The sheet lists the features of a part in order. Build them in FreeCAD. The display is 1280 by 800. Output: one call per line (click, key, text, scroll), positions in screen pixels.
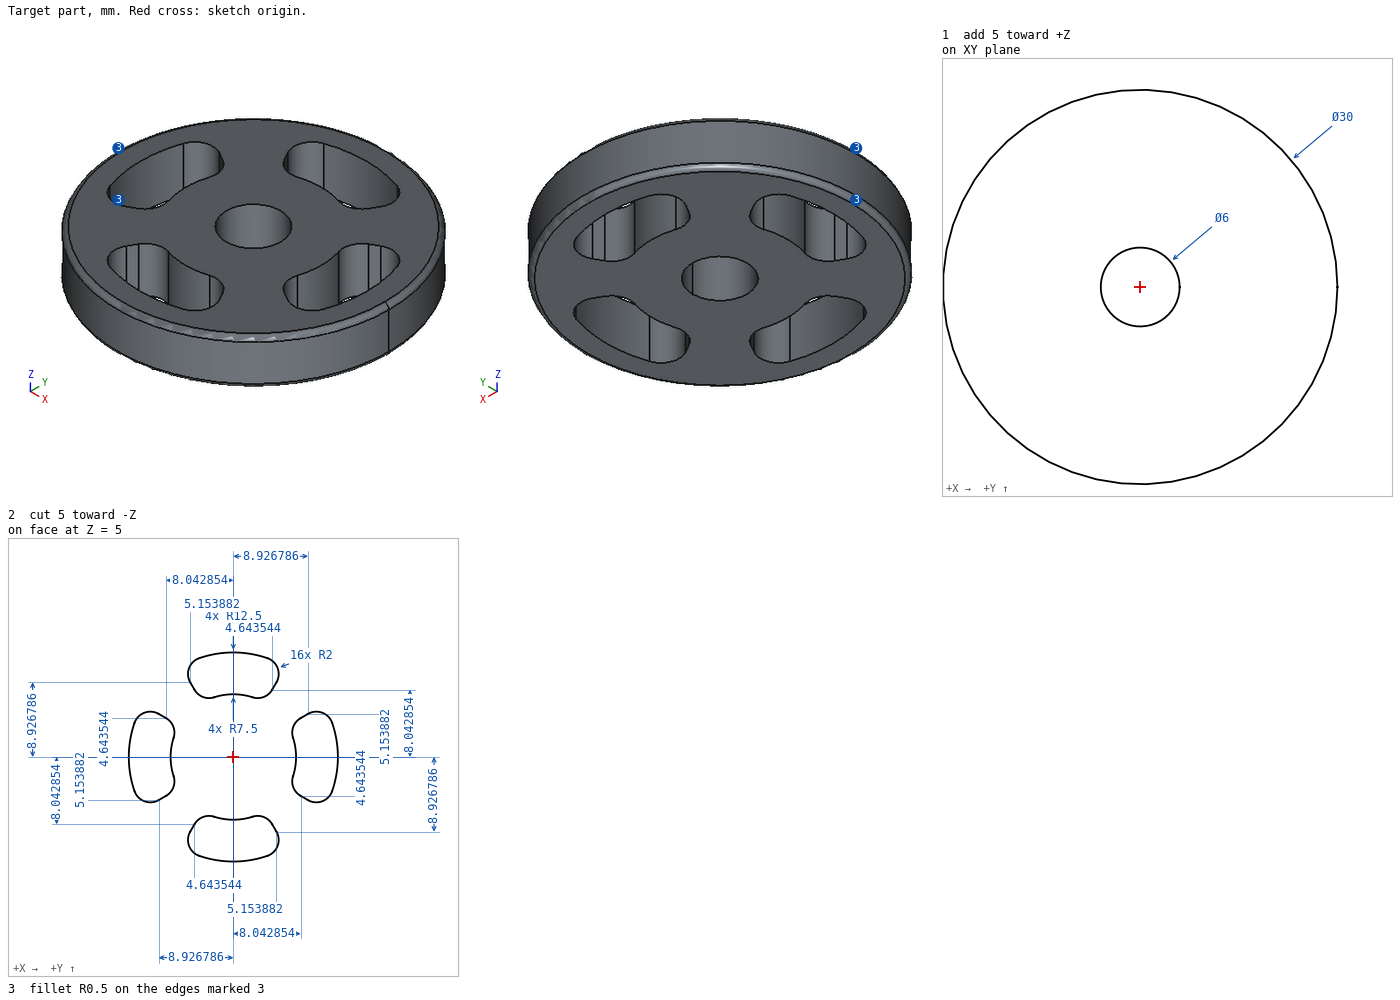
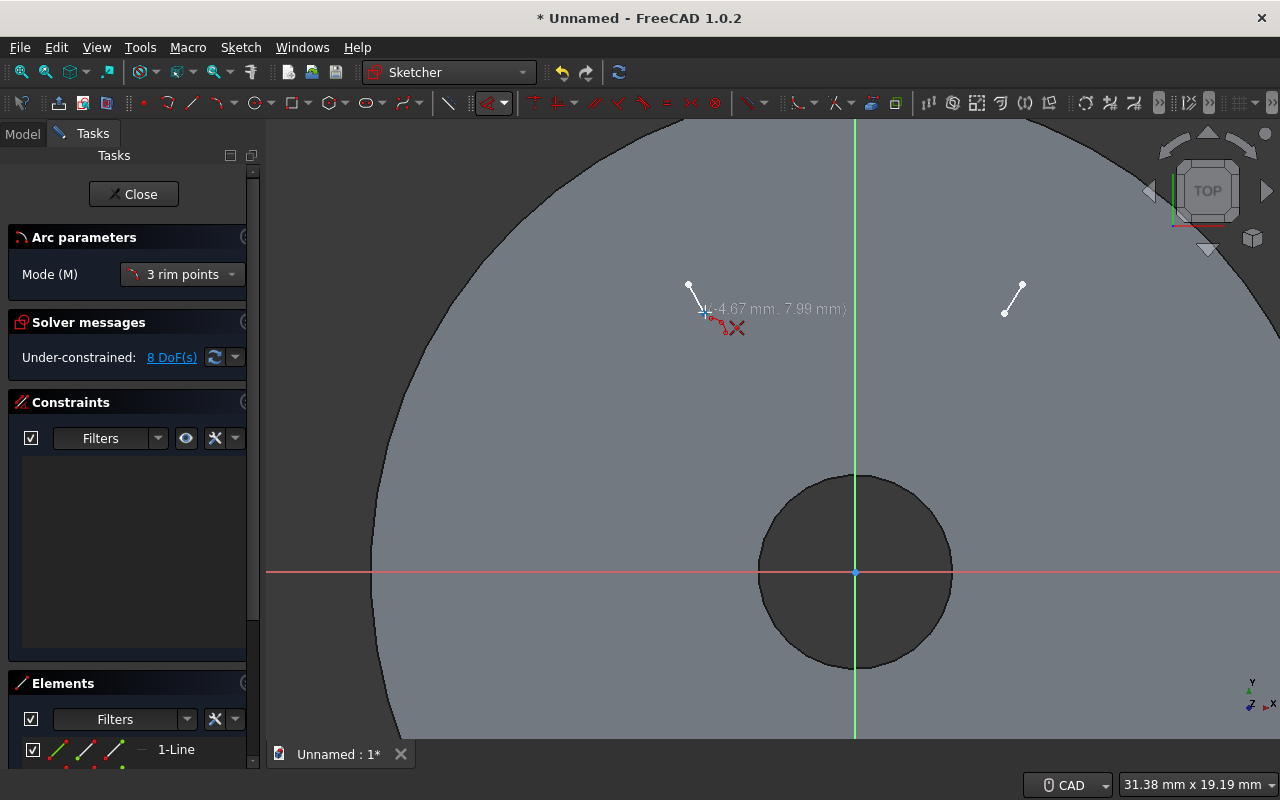
click(704, 314)
click(781, 341)
click(738, 340)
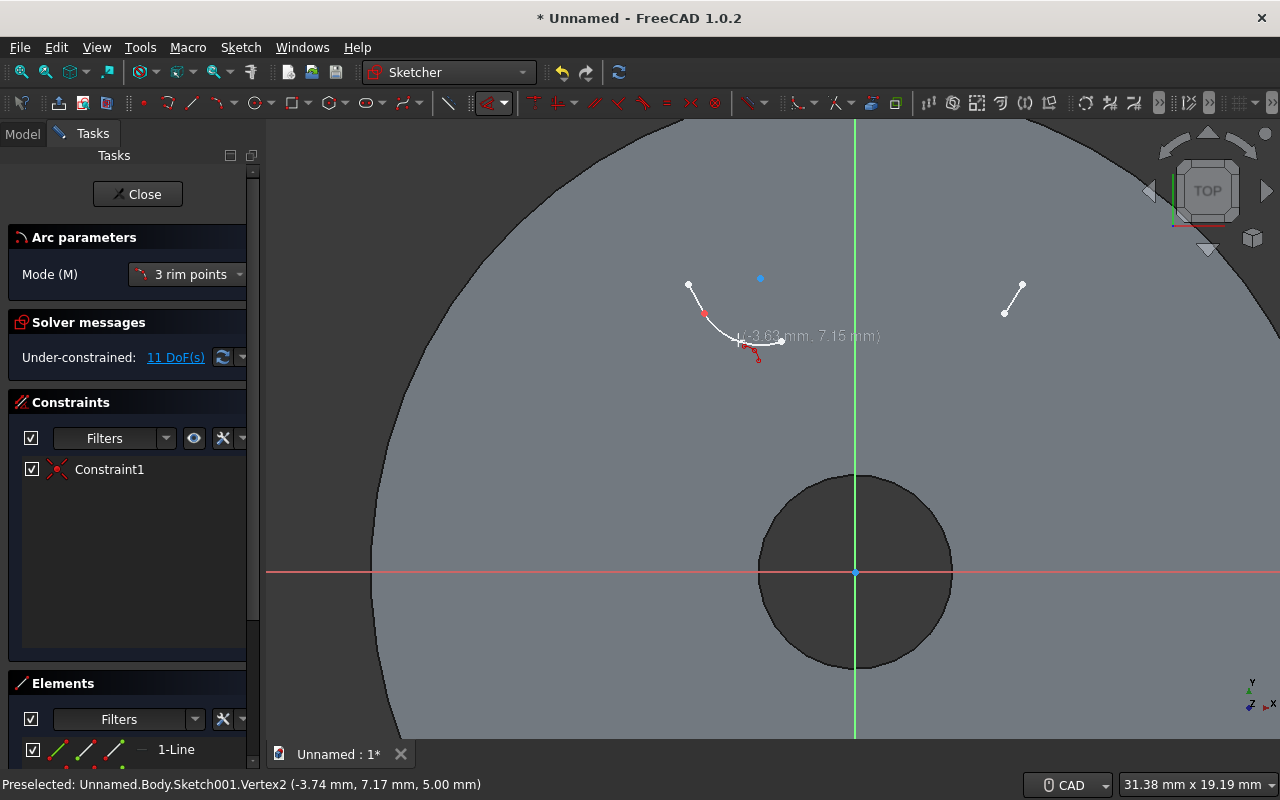
click(781, 342)
click(930, 341)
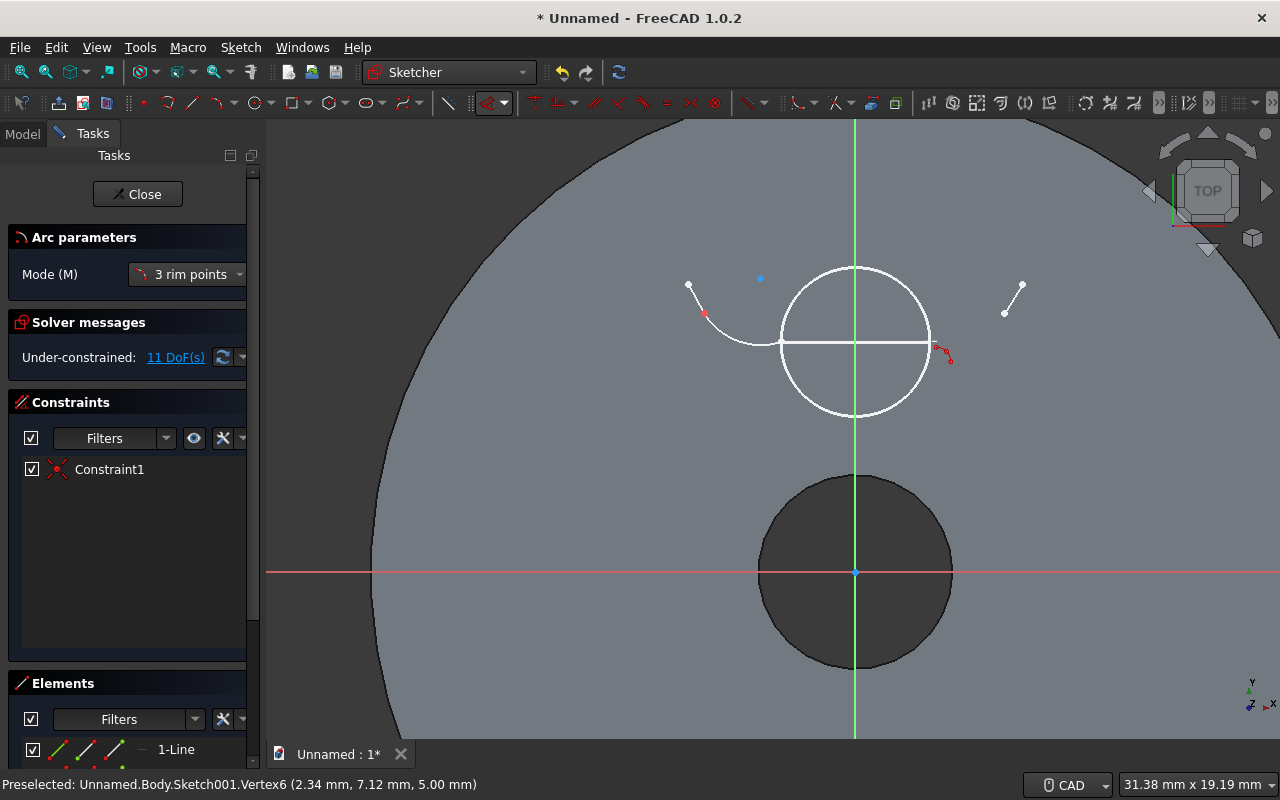
scroll(871, 330, up, 2)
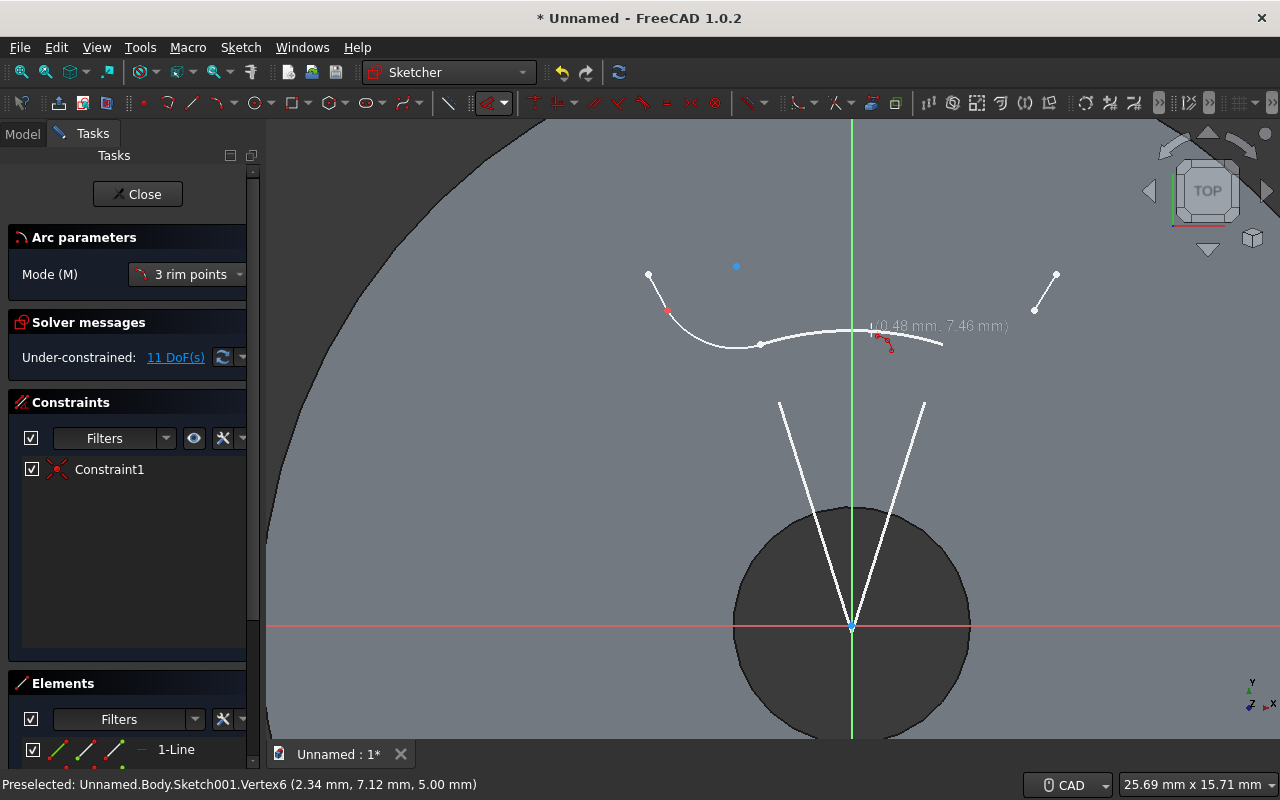
click(870, 330)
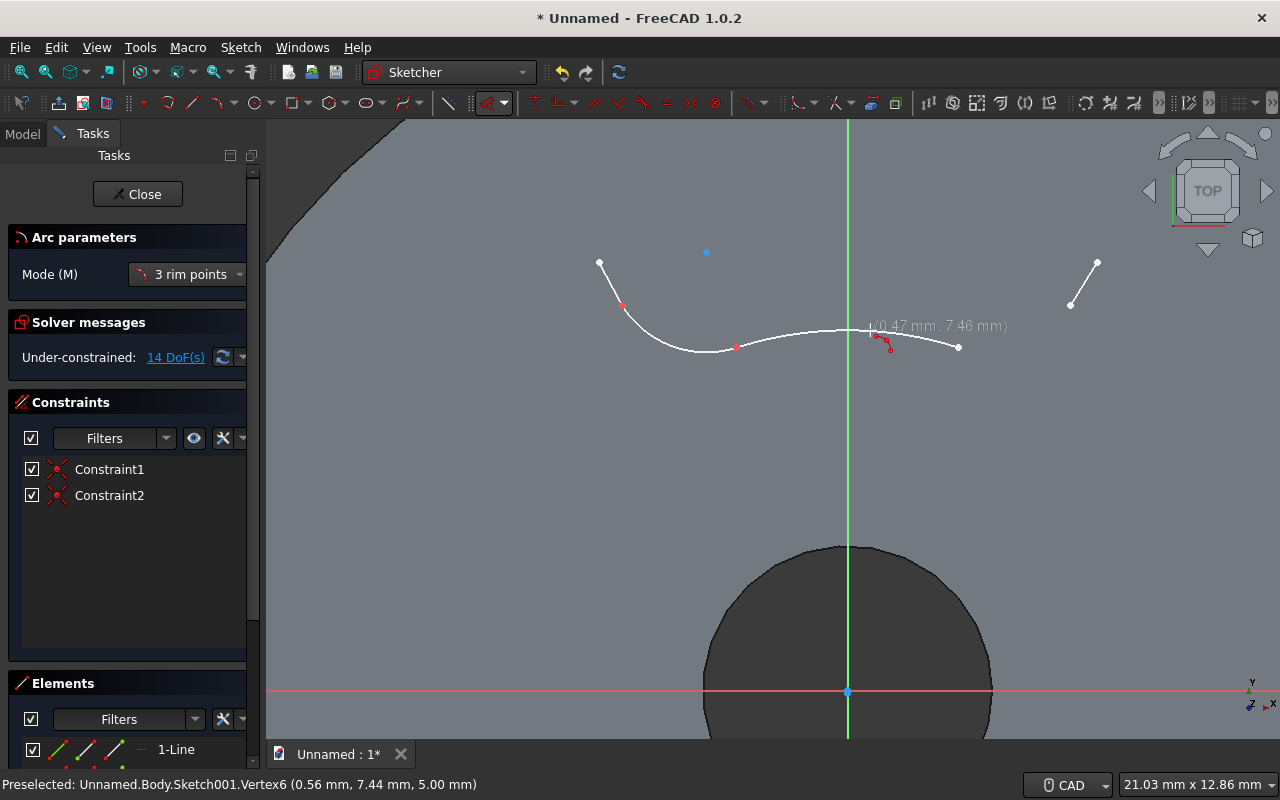
click(959, 348)
click(1070, 306)
click(1023, 345)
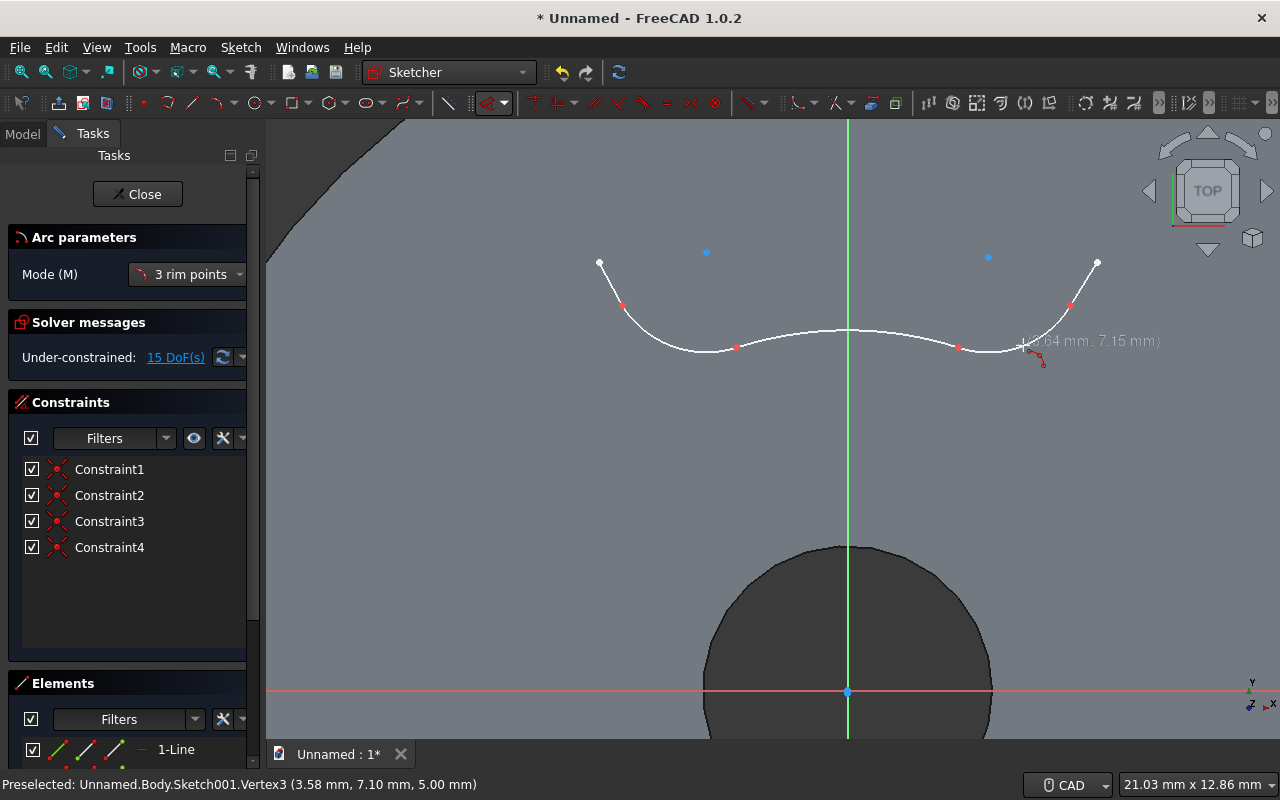
click(1097, 263)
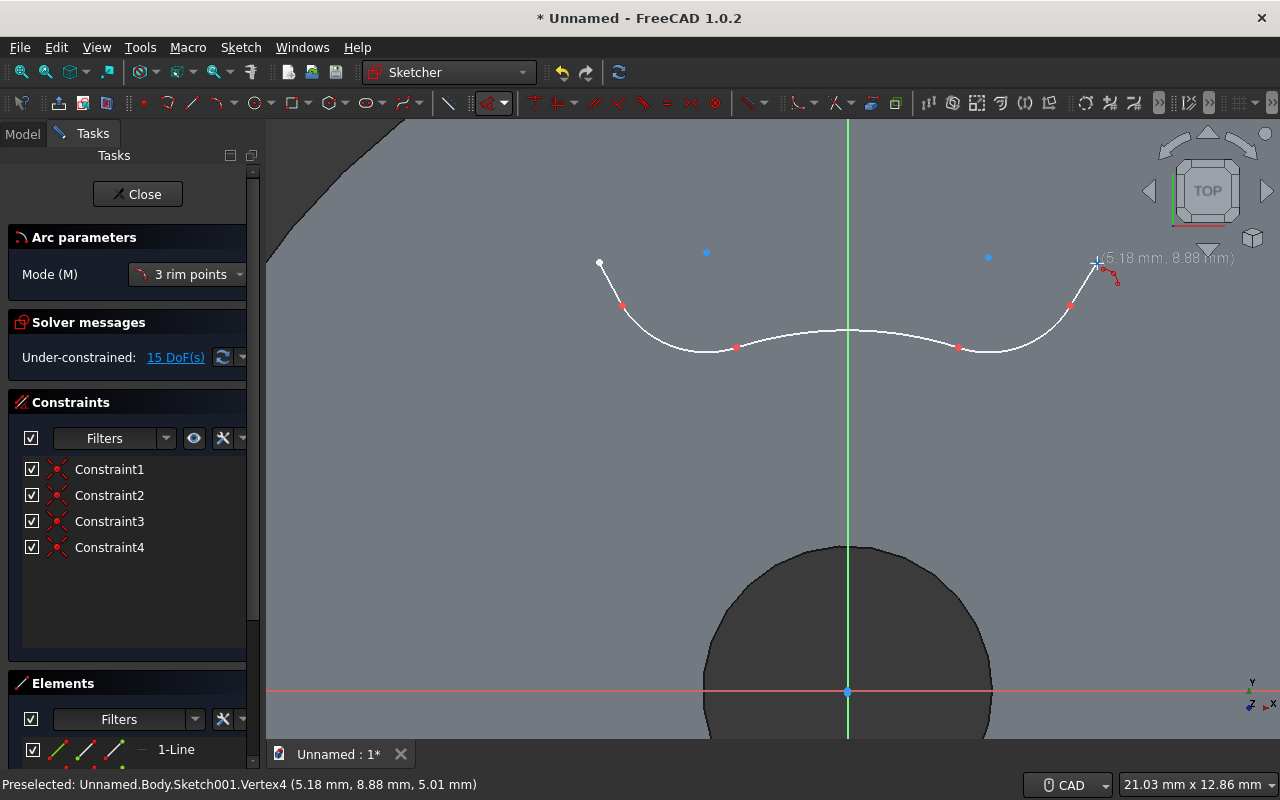
scroll(643, 316, down, 6)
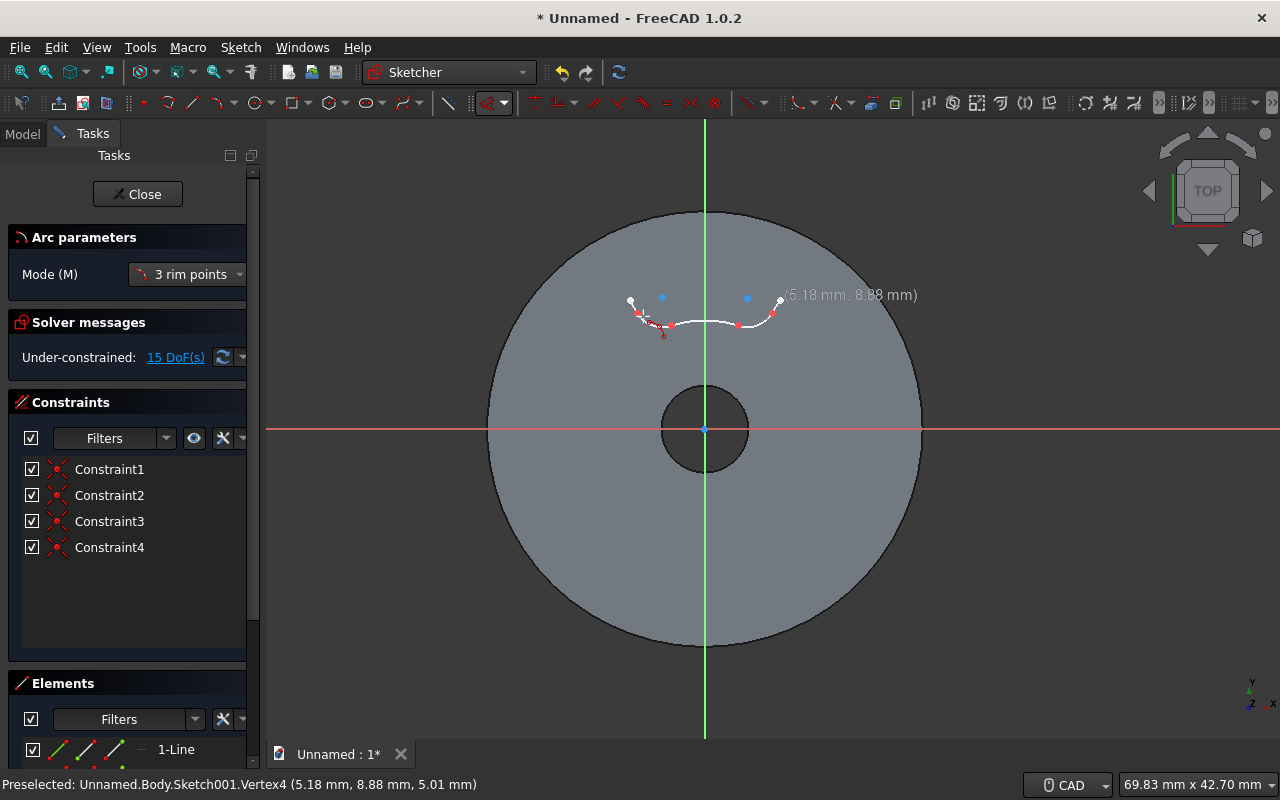
click(764, 258)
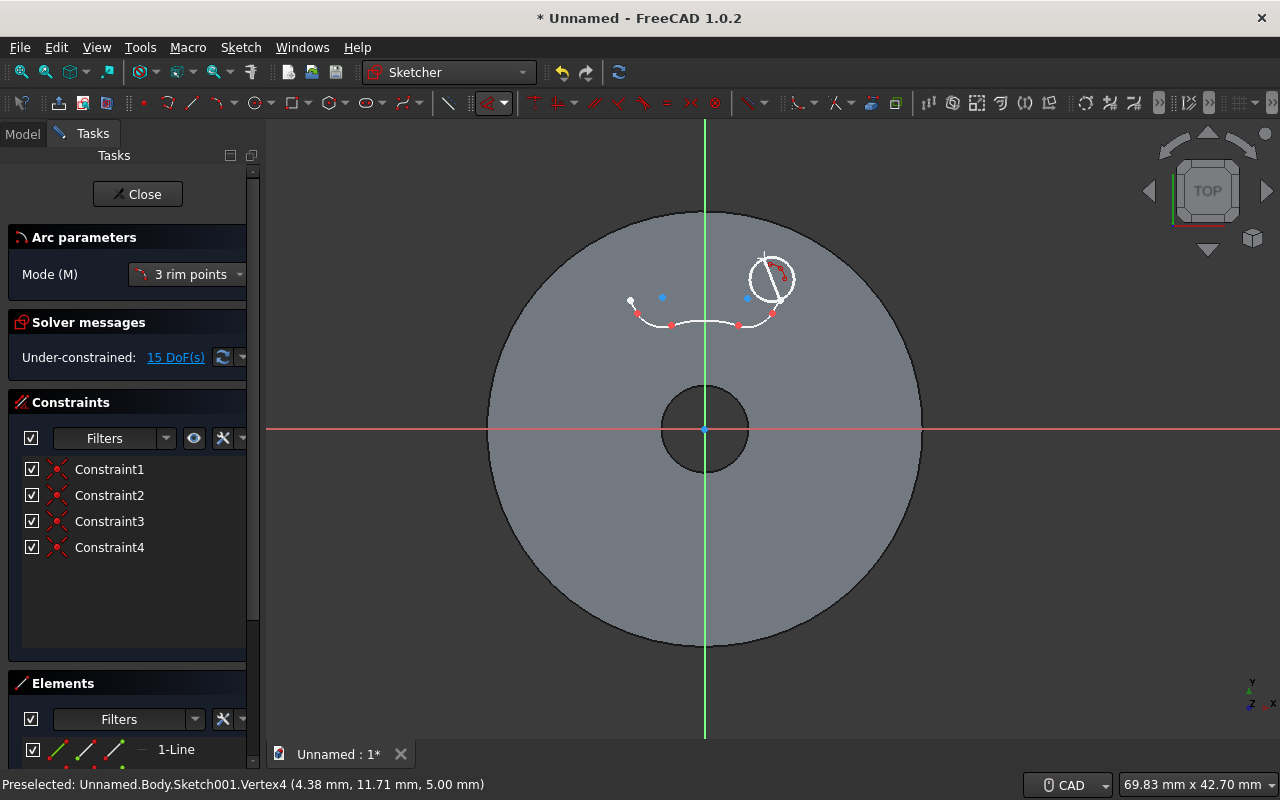
scroll(782, 275, up, 3)